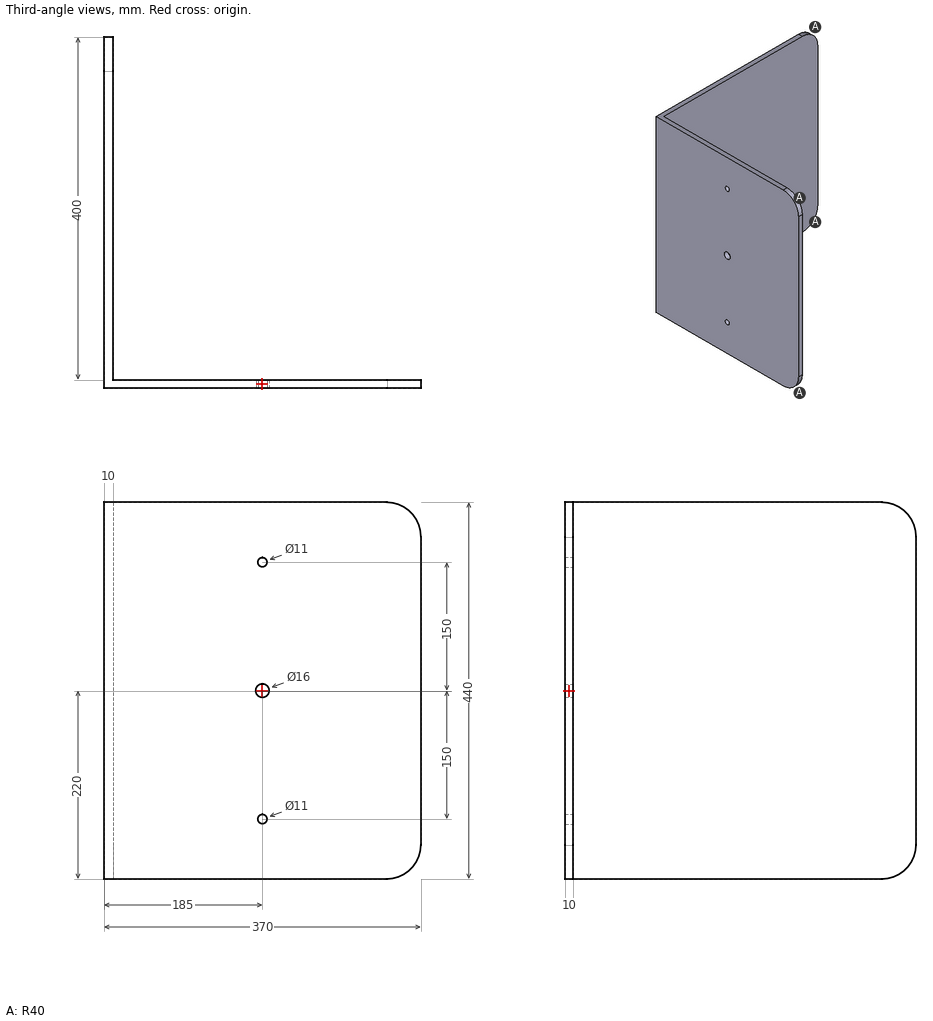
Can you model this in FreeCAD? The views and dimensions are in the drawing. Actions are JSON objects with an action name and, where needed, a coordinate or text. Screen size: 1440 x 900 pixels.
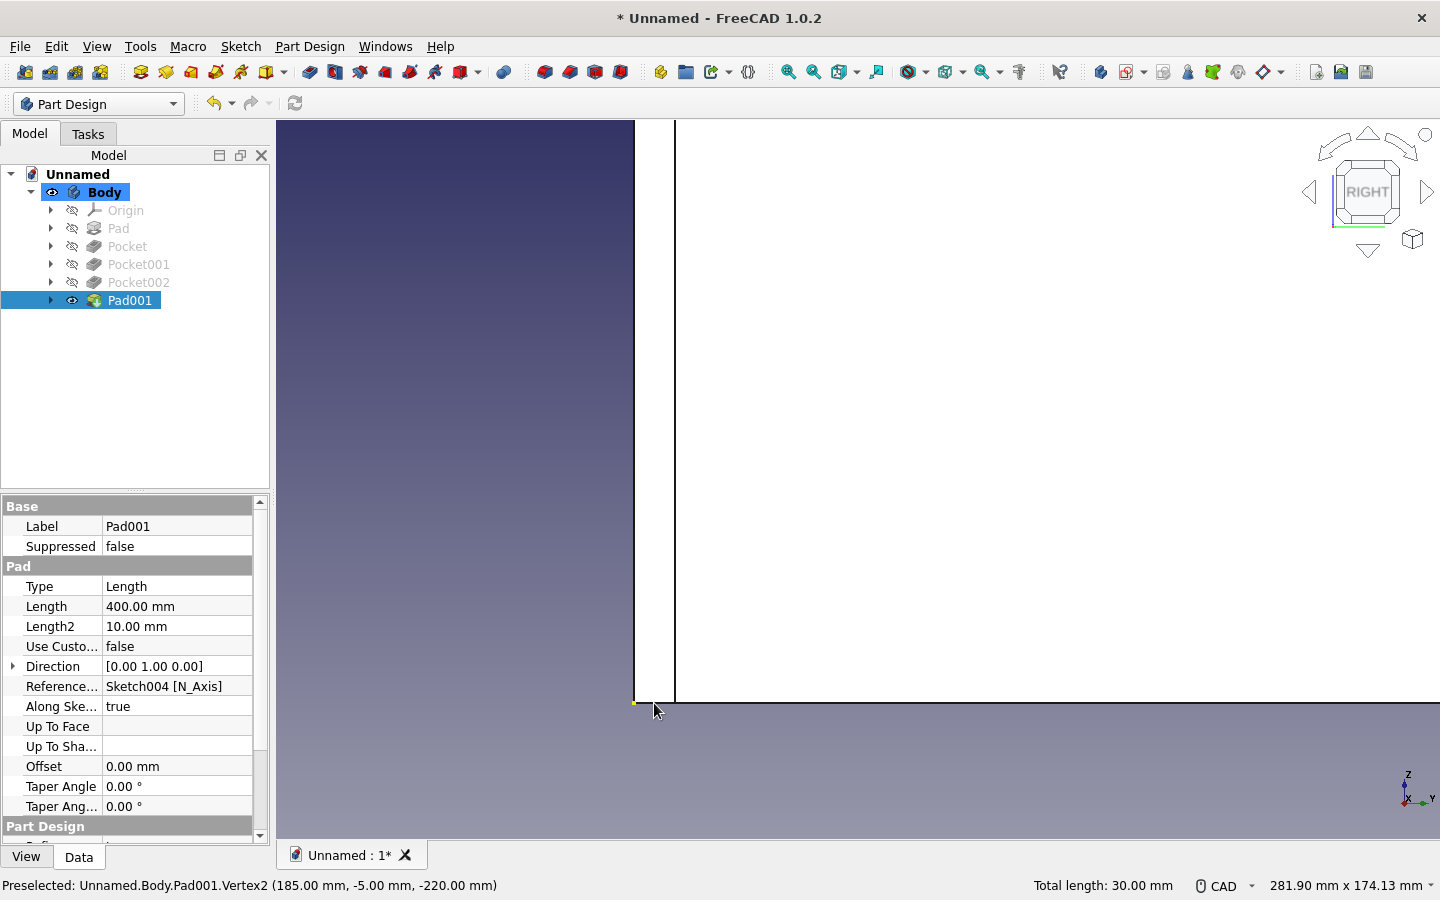
{"action": "left_click", "coordinate": [654, 702], "text": "ctrl"}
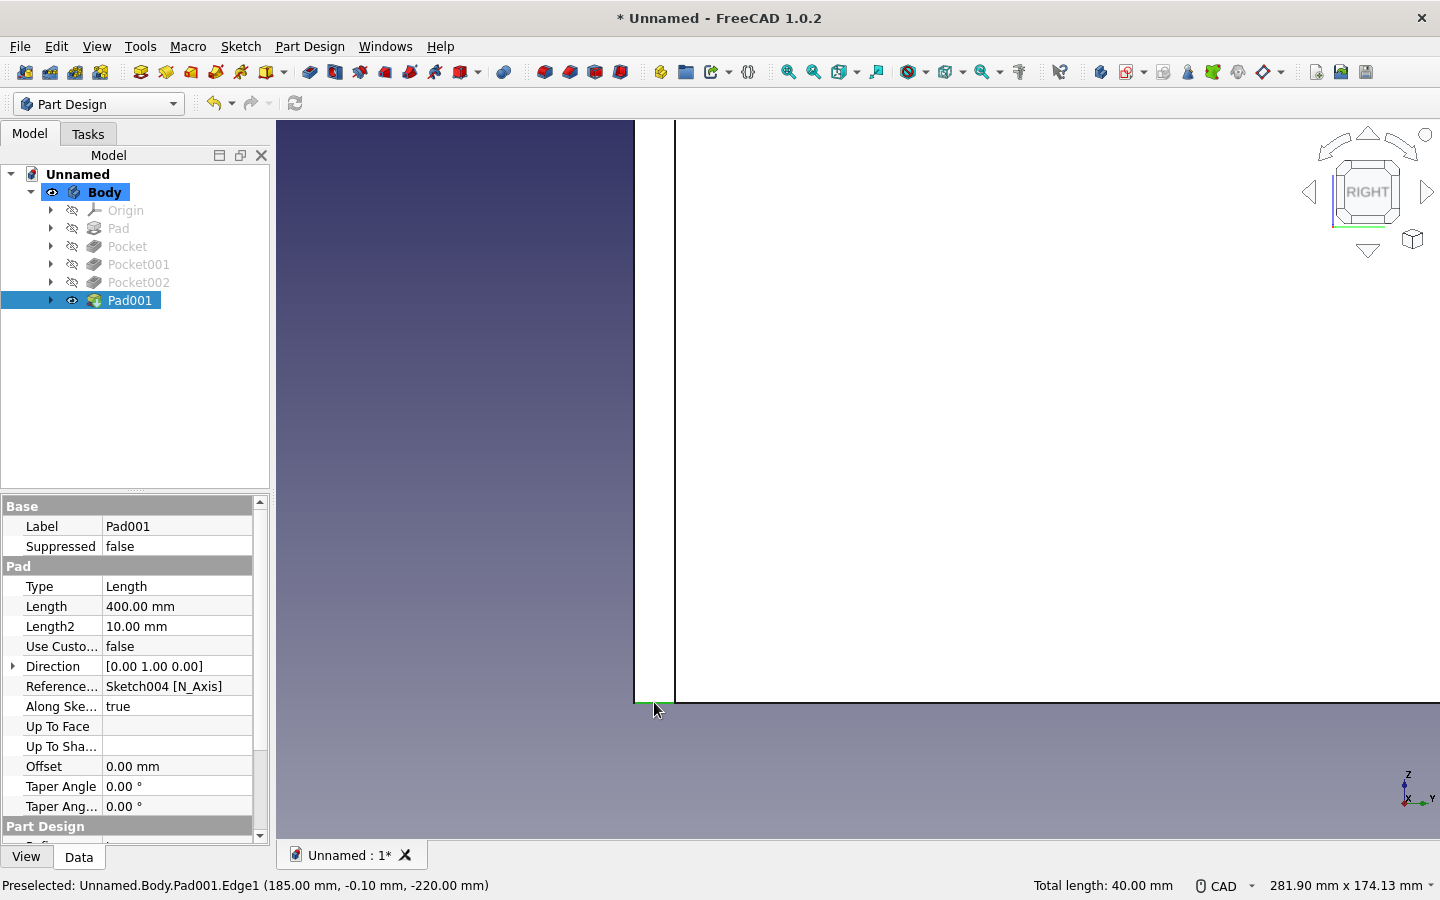
{"action": "left_click", "coordinate": [545, 72]}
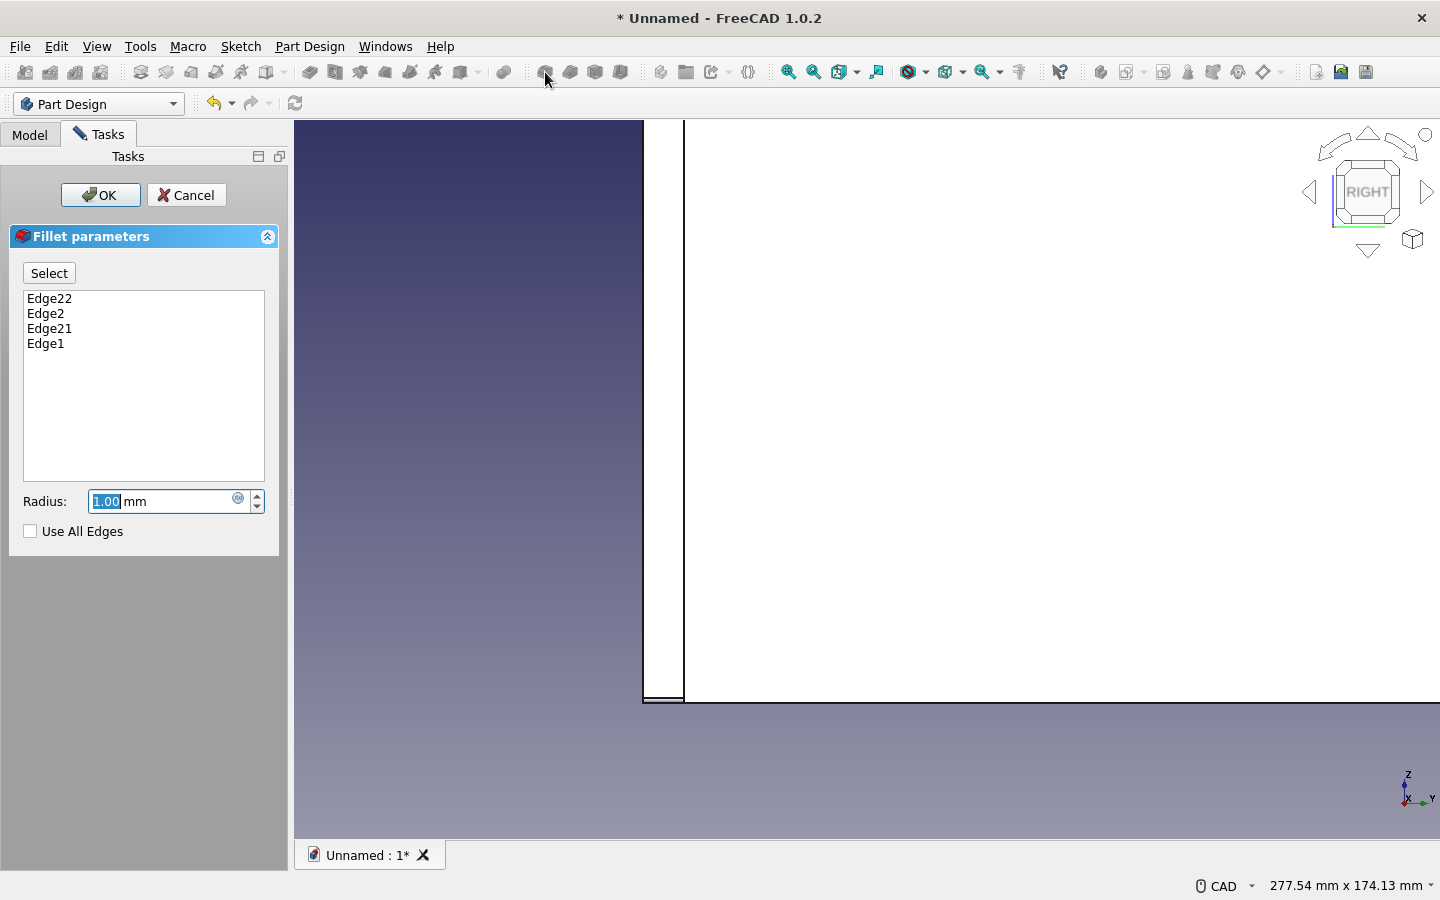
{"action": "type", "text": "40"}
{"action": "key", "text": "Tab"}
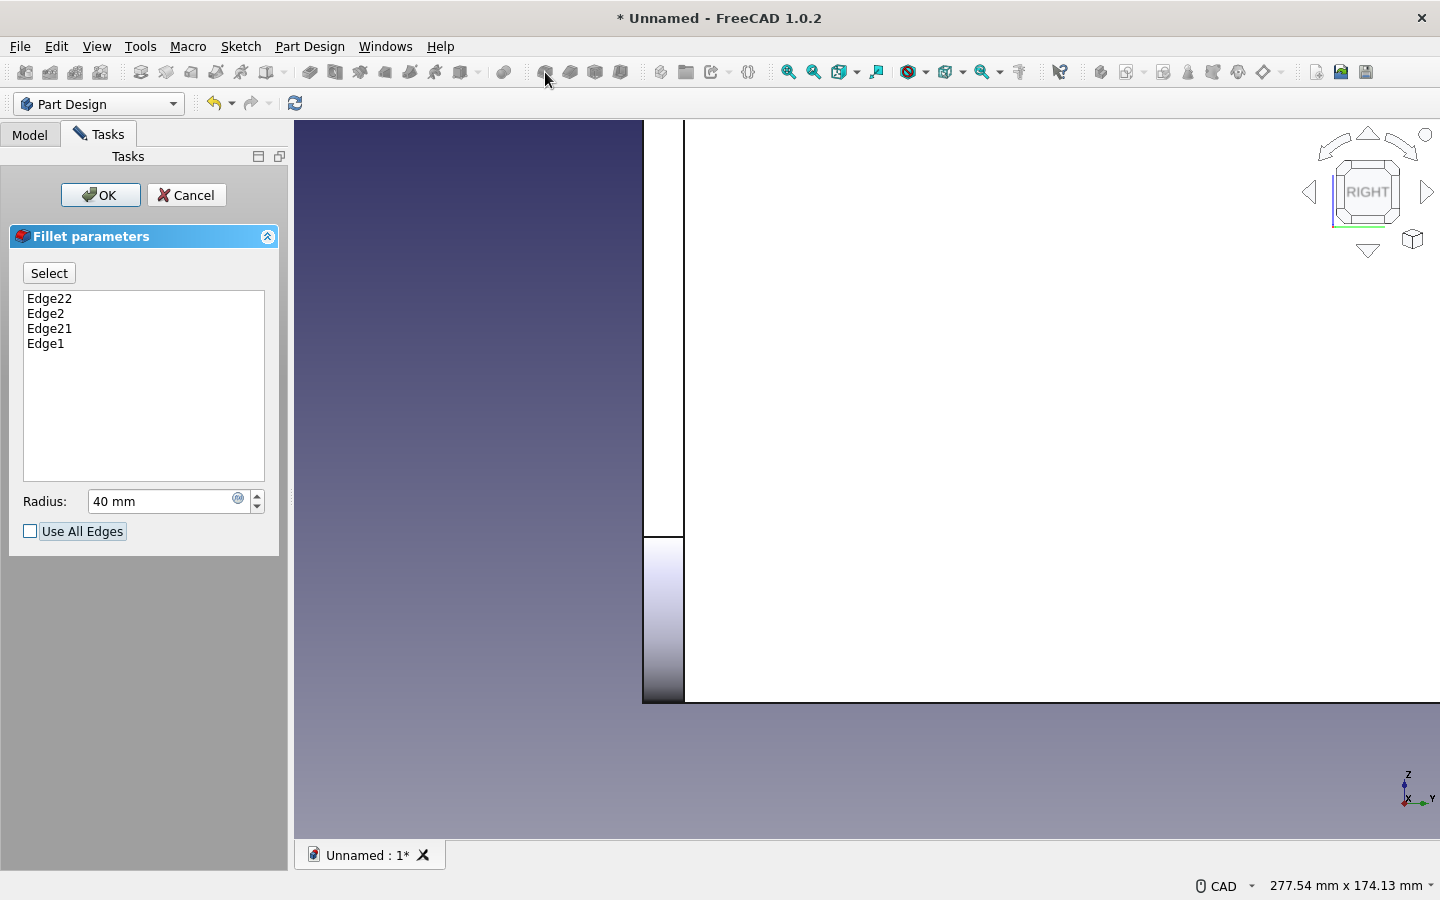
{"action": "left_click", "coordinate": [101, 195]}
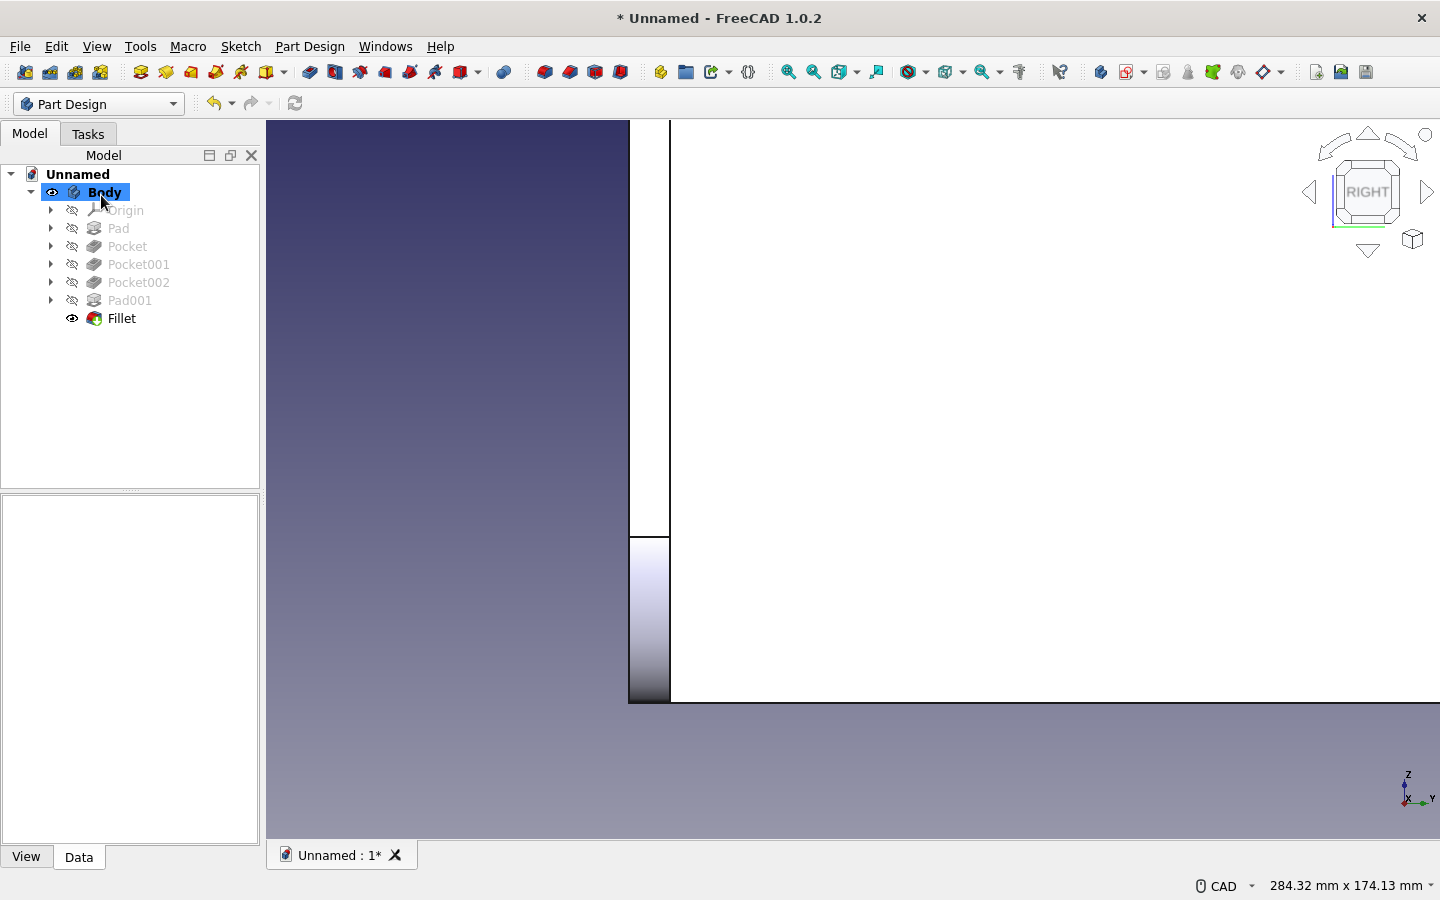
{"action": "key", "text": "0"}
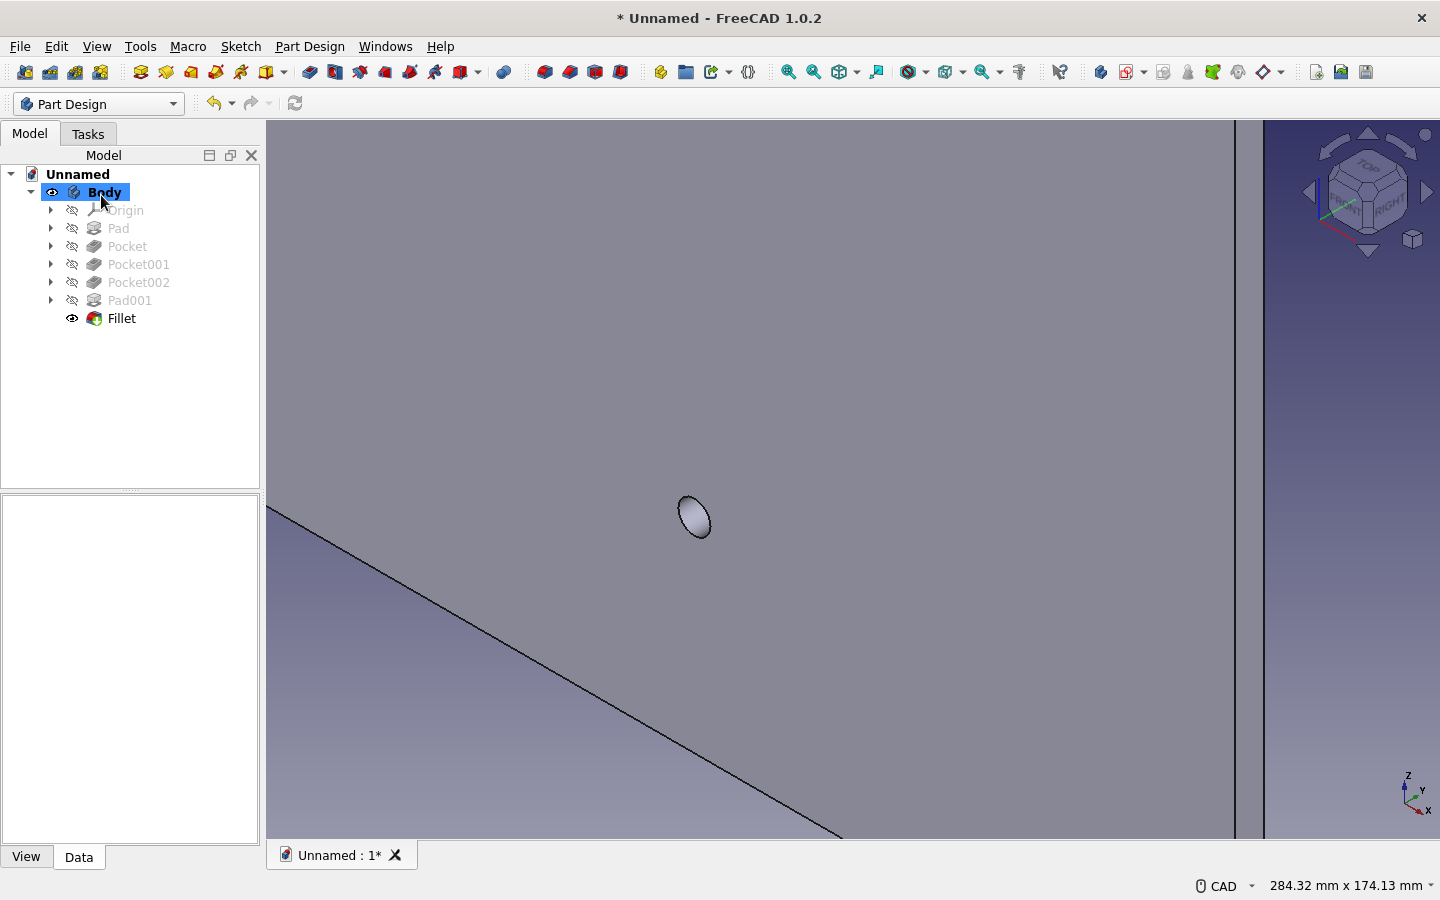
{"action": "left_click", "coordinate": [789, 72]}